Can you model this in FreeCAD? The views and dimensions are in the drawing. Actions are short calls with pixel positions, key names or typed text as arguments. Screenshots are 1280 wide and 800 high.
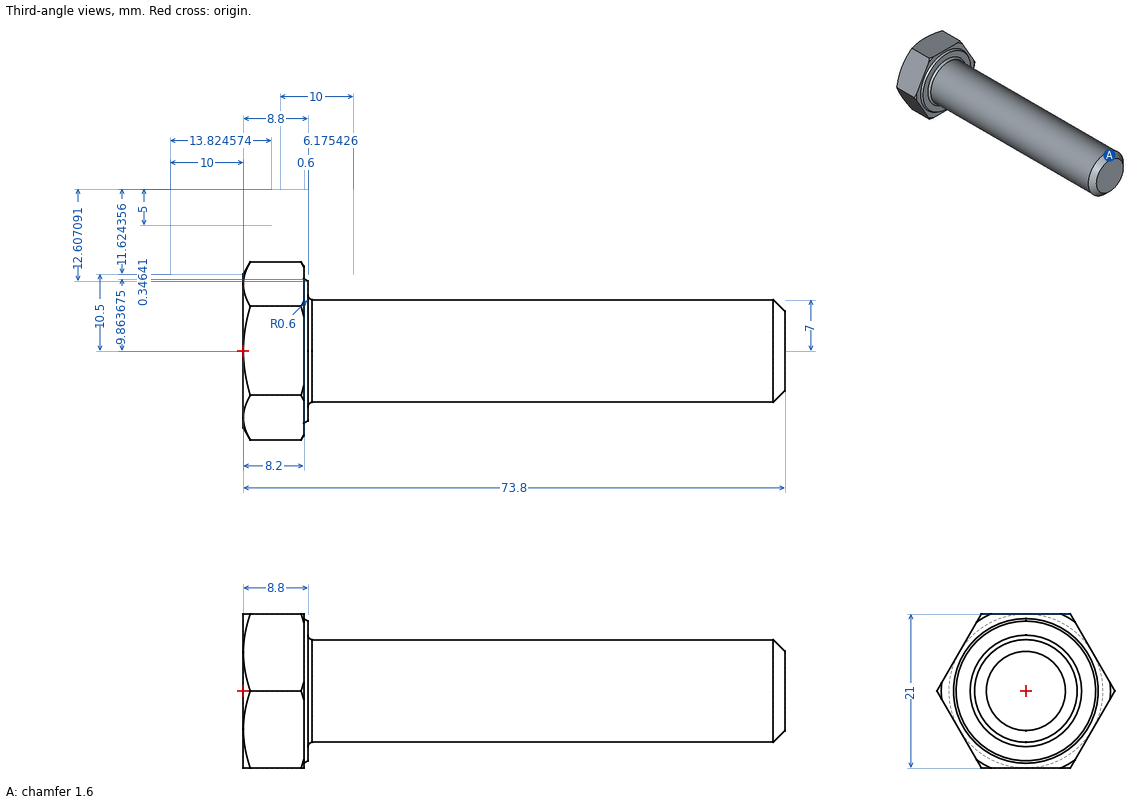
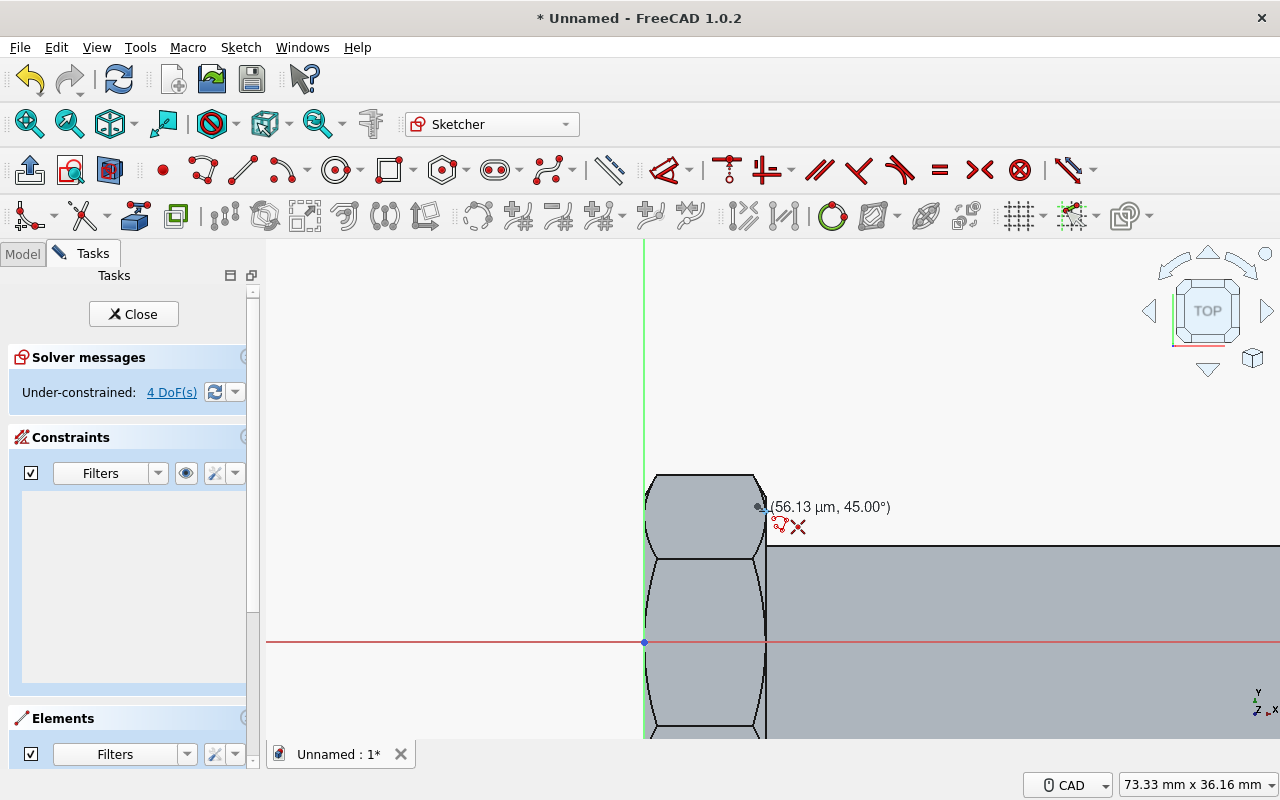
click(766, 336)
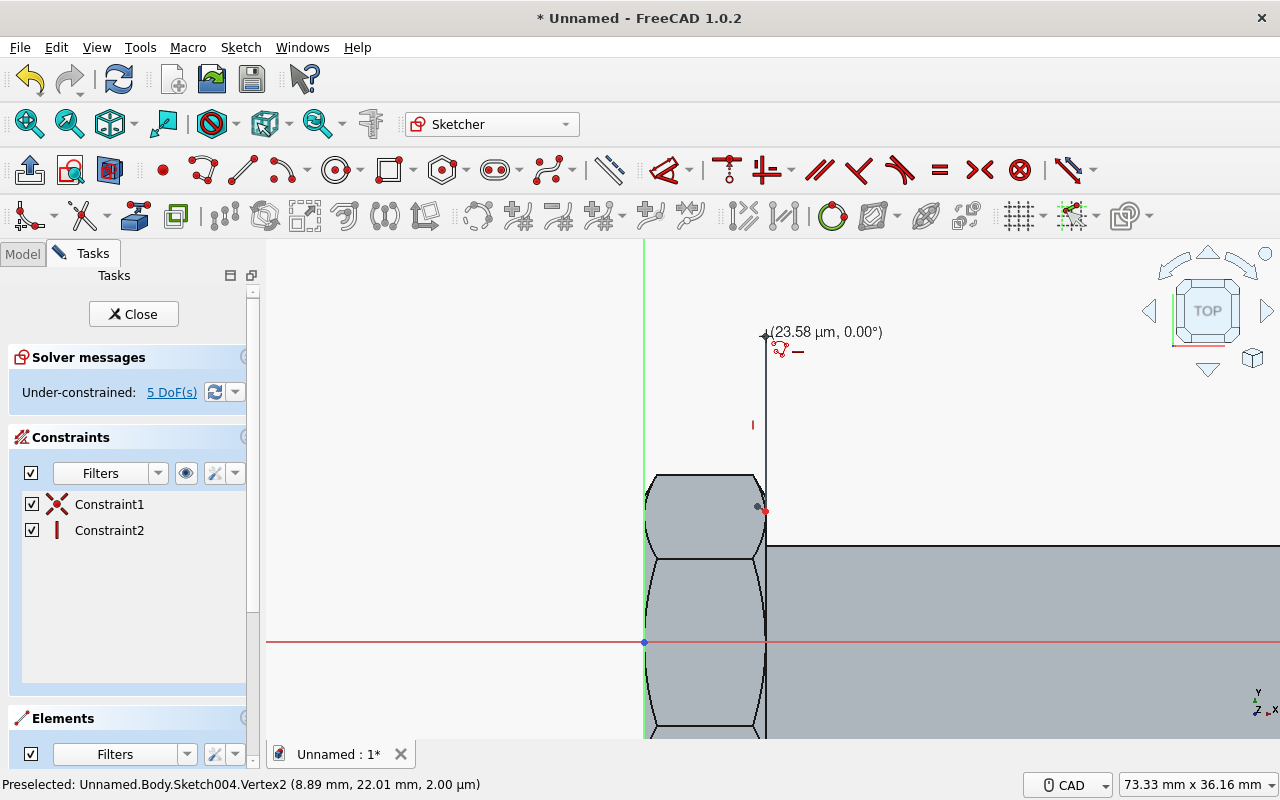
scroll(757, 336, up, 4)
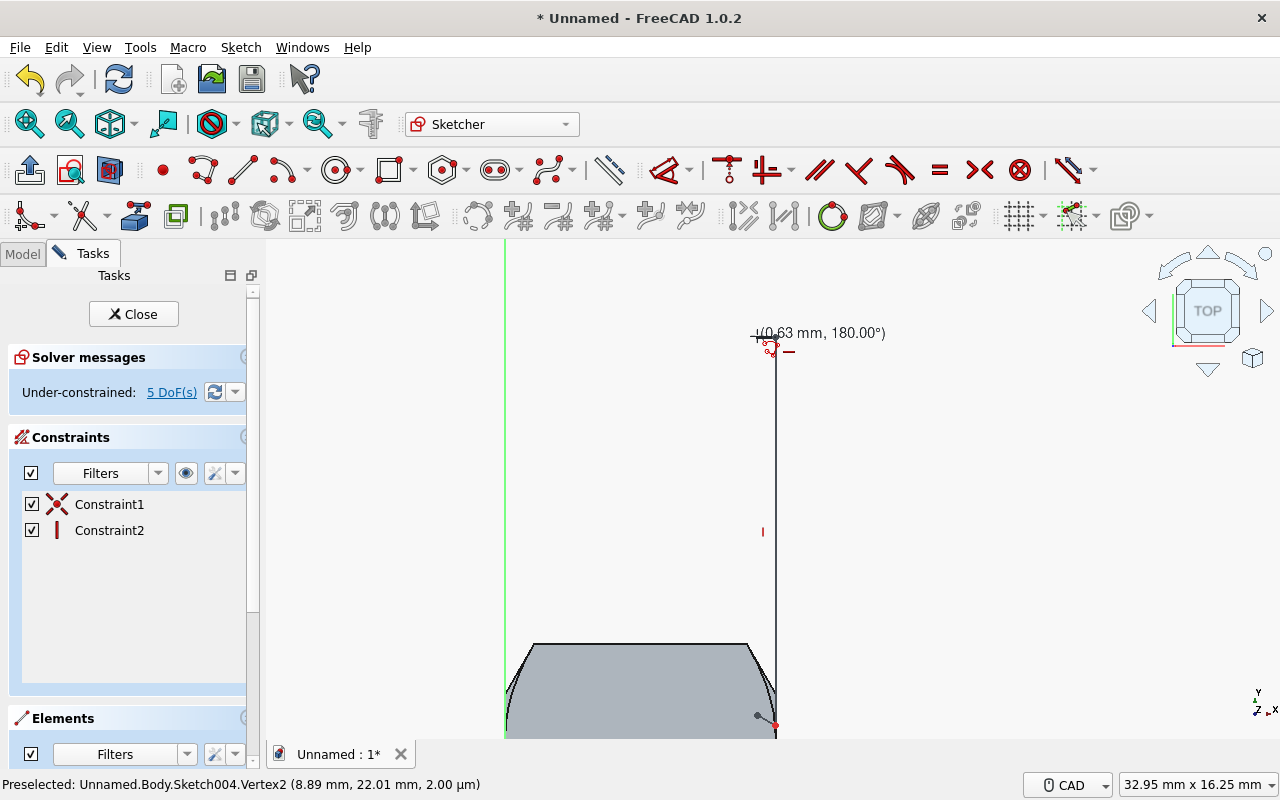
click(757, 336)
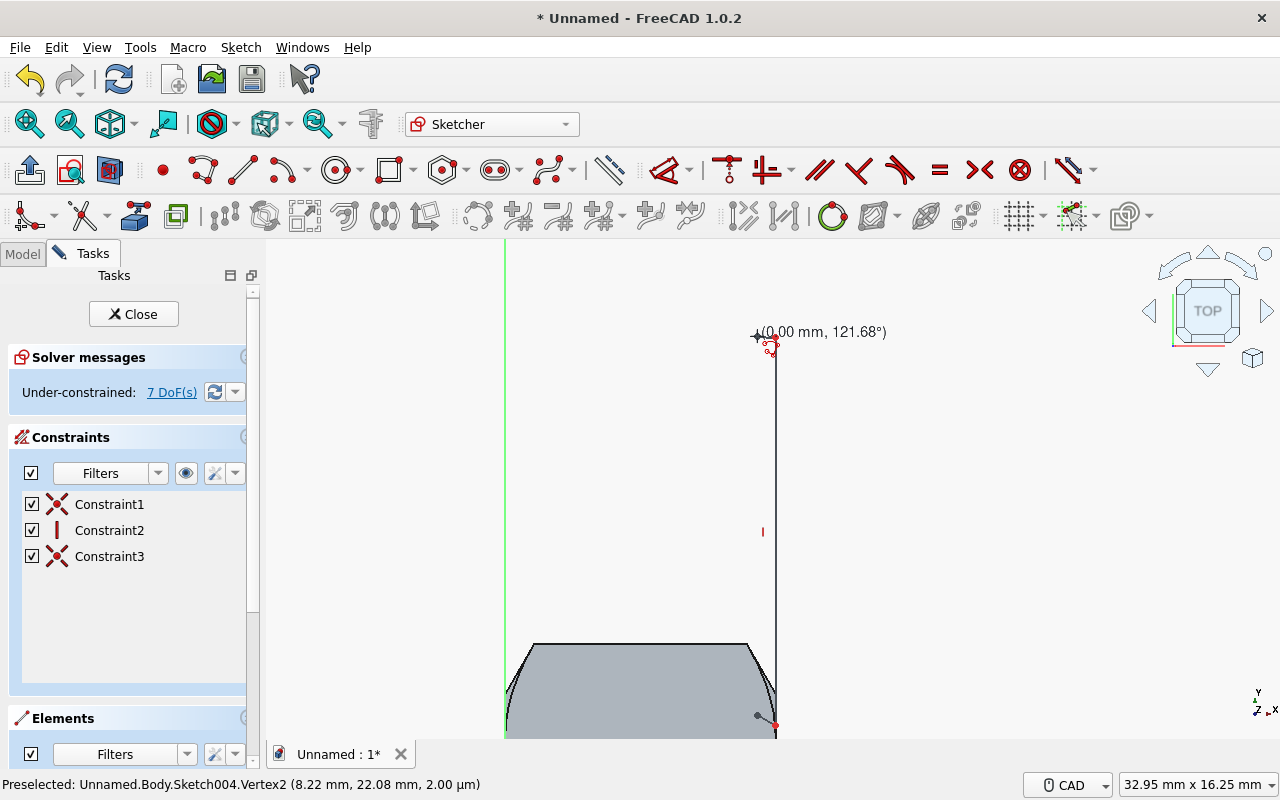
scroll(757, 336, down, 4)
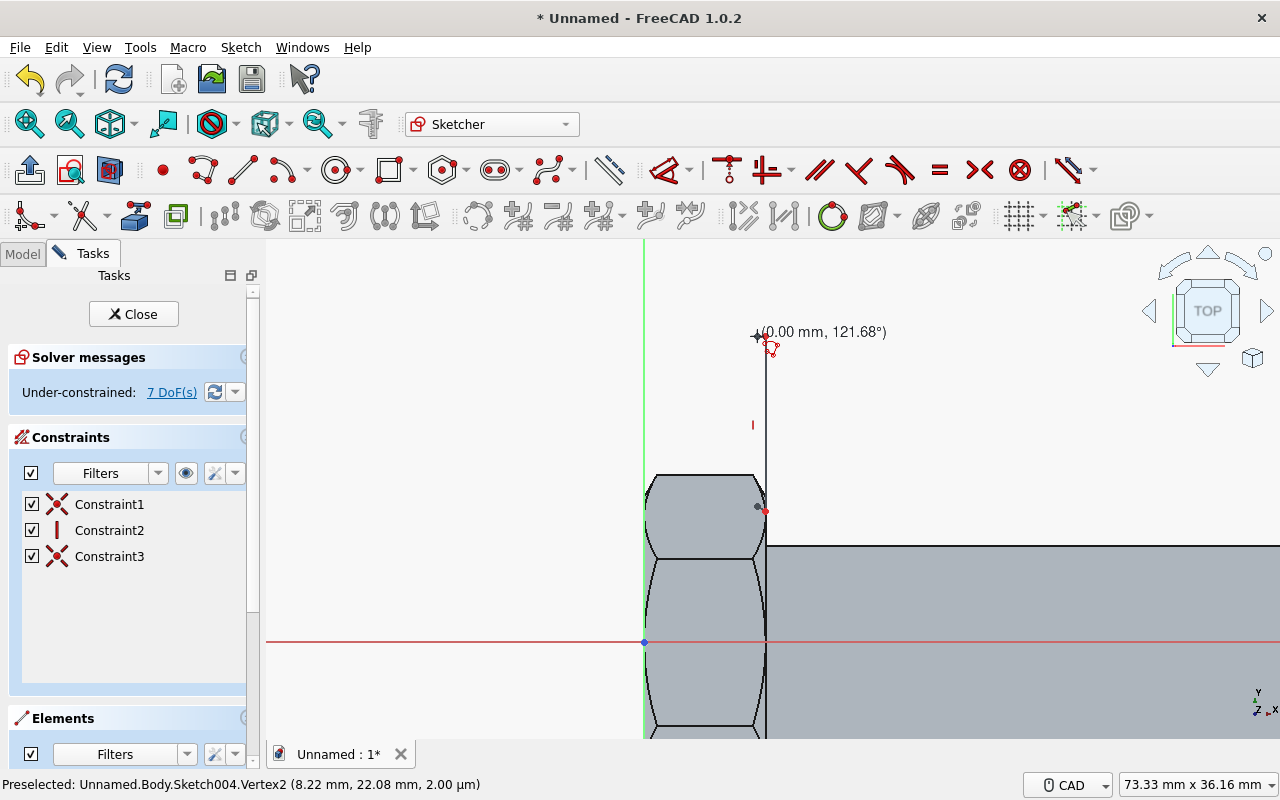
scroll(757, 506, up, 6)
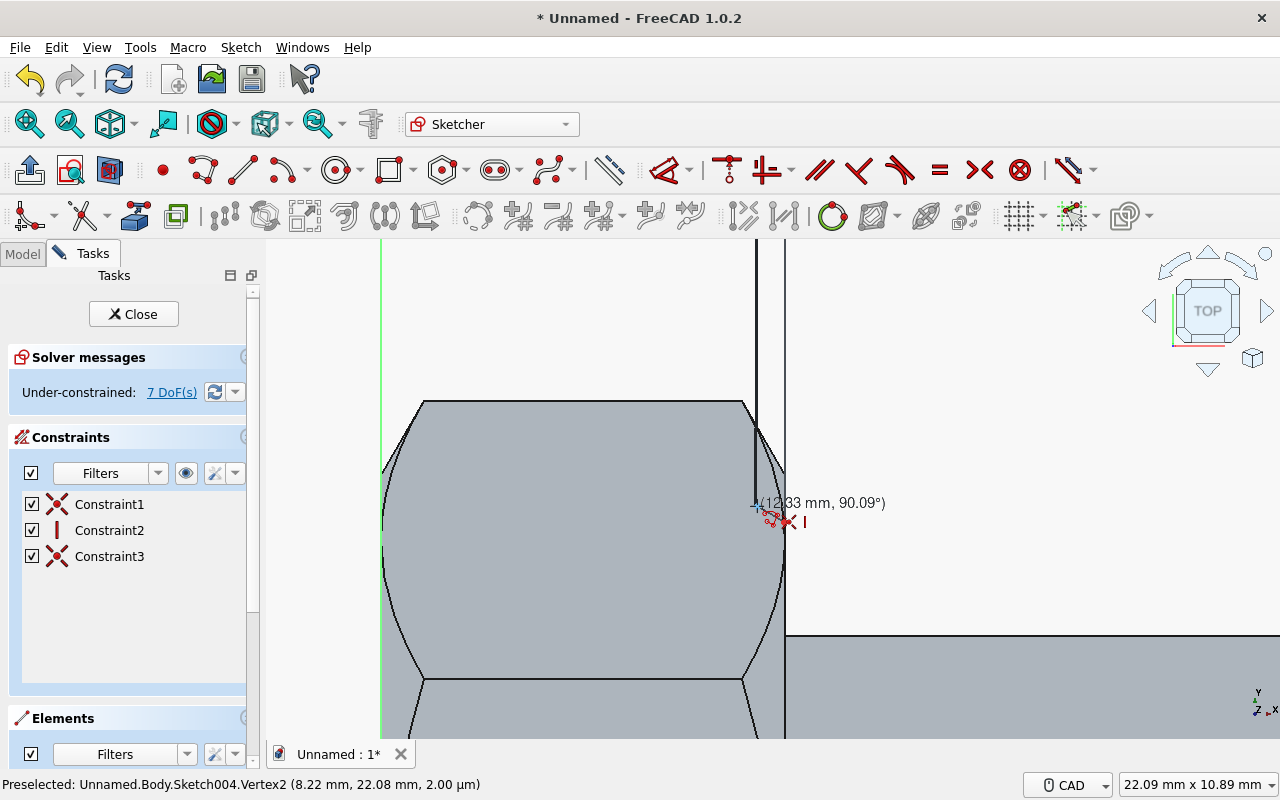
click(757, 506)
key(Escape)
key(Escape)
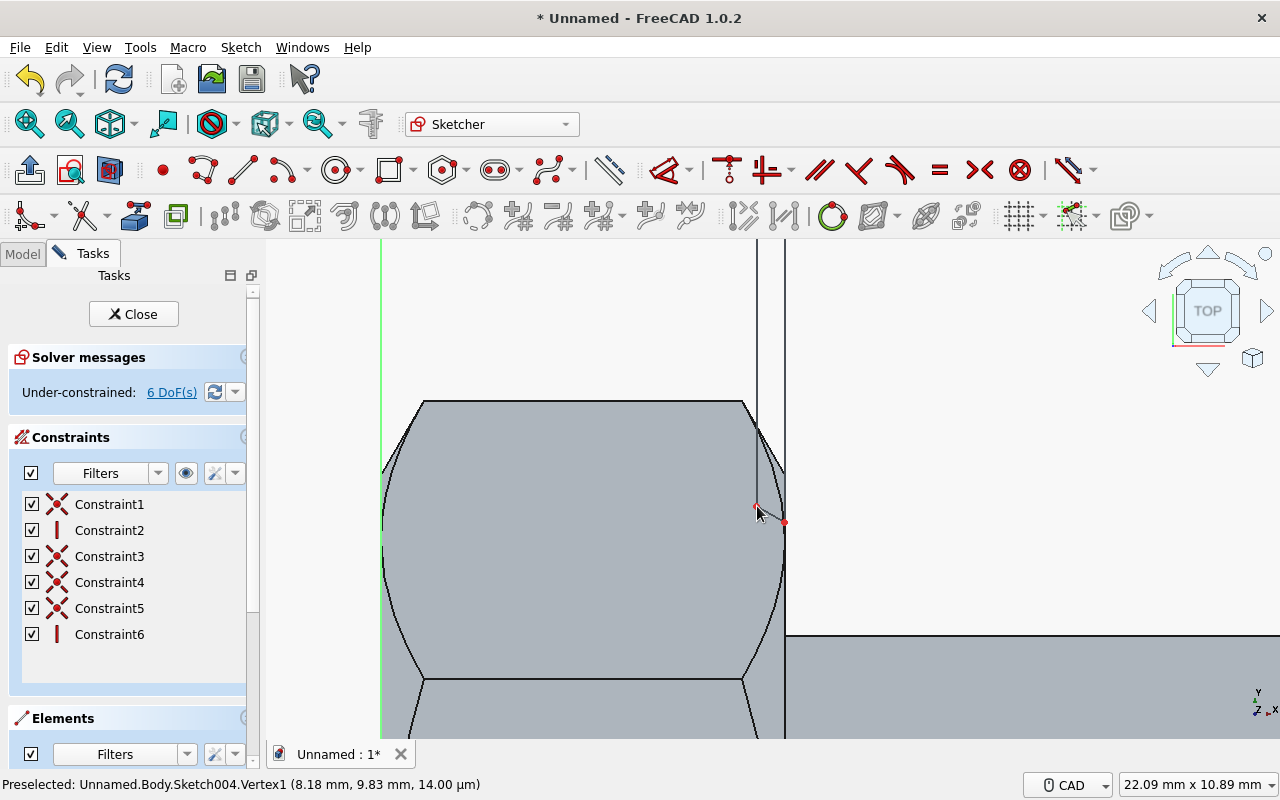
scroll(757, 506, down, 6)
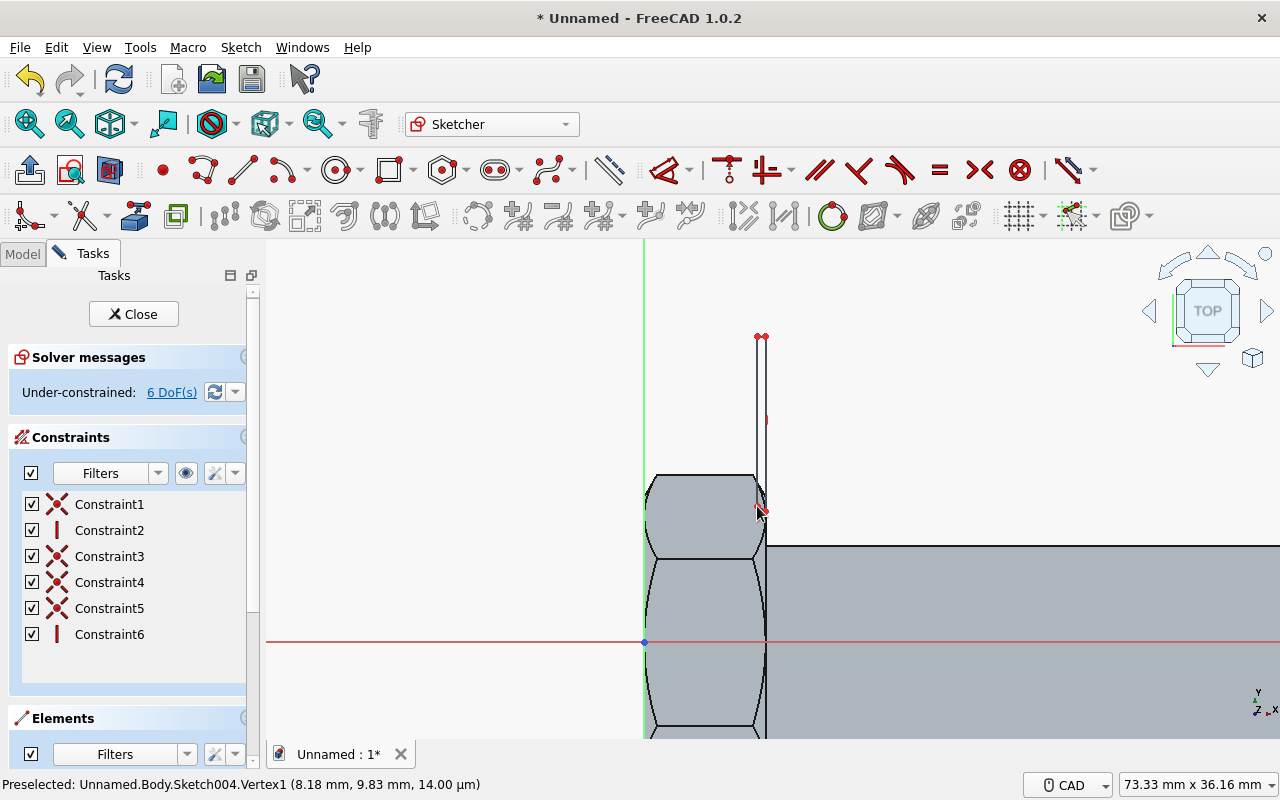
scroll(762, 337, up, 8)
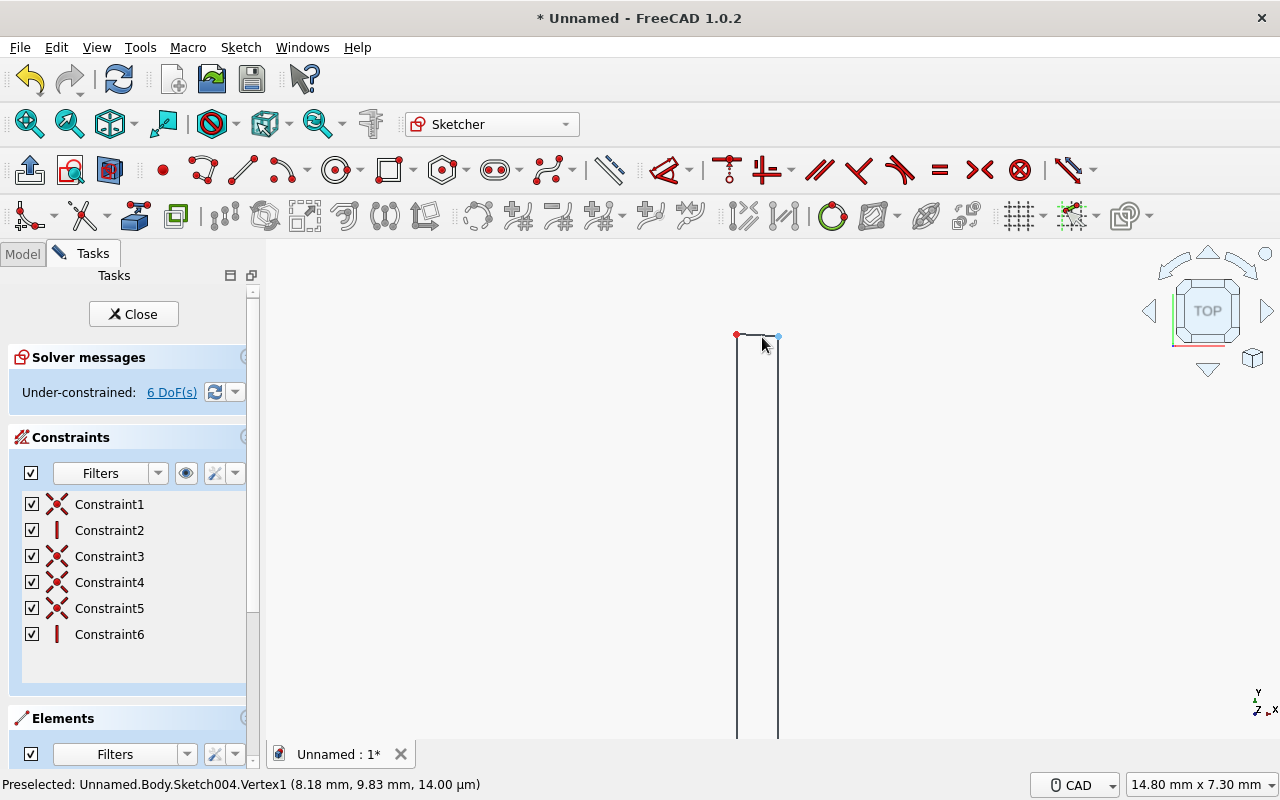
click(762, 335)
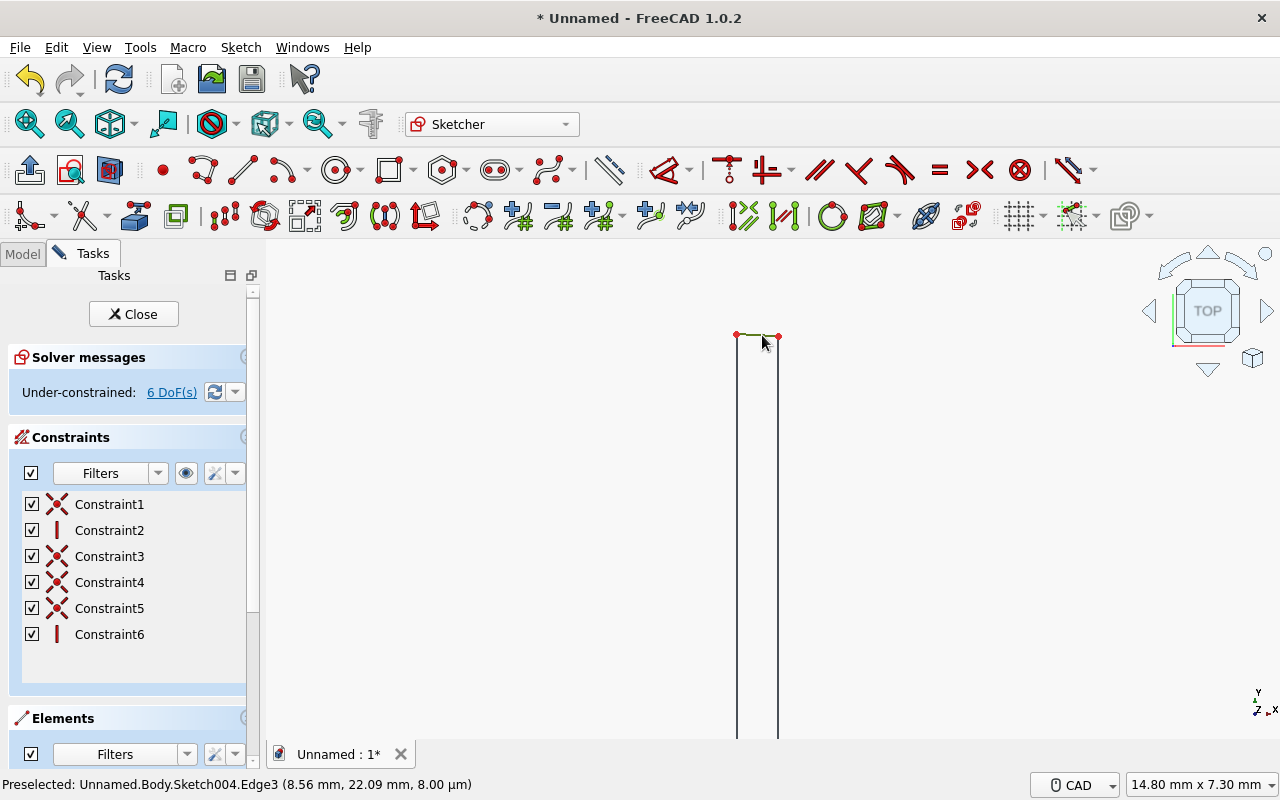
click(794, 170)